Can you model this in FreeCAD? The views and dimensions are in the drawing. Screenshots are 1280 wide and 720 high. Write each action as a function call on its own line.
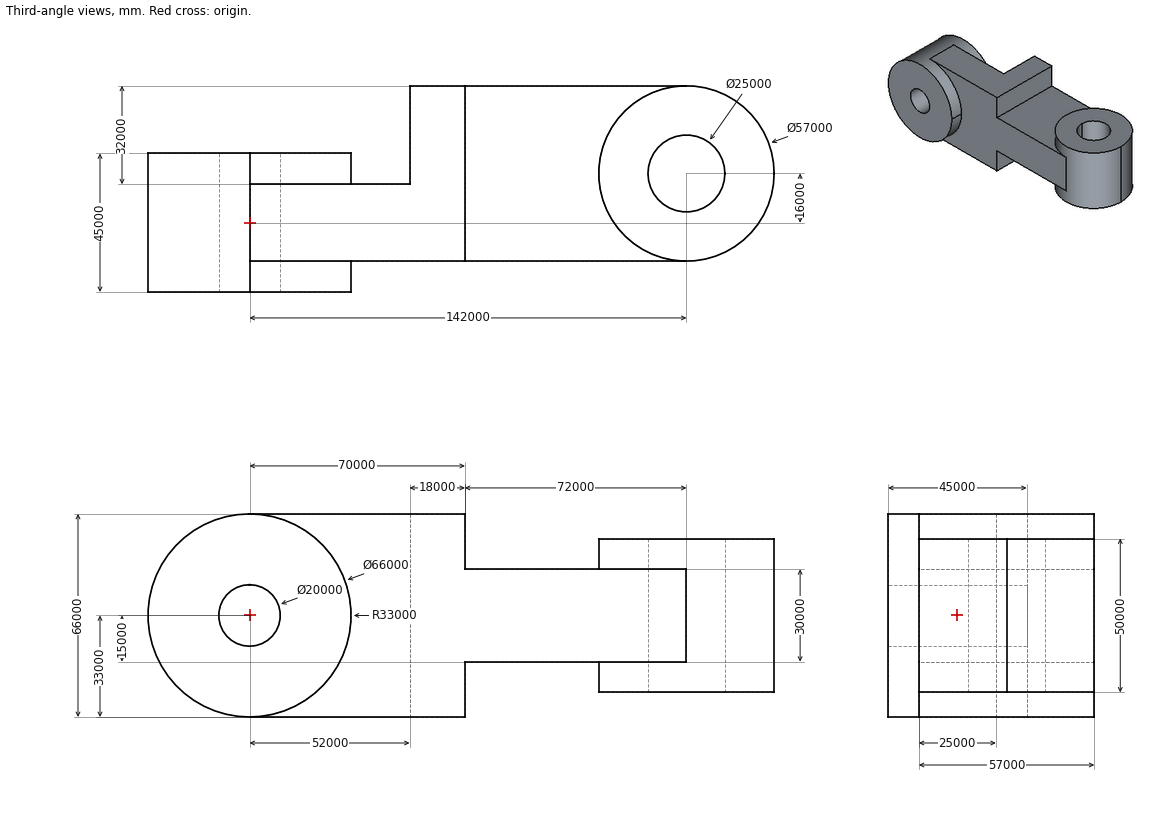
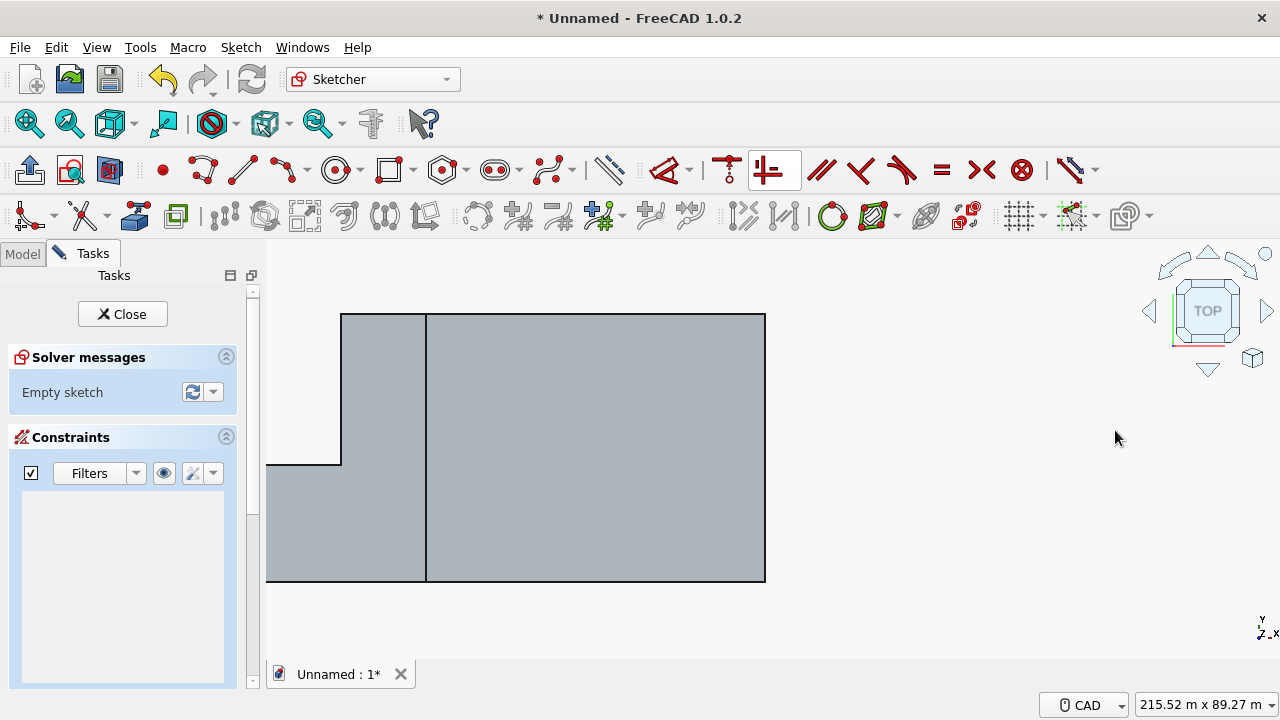
click(336, 170)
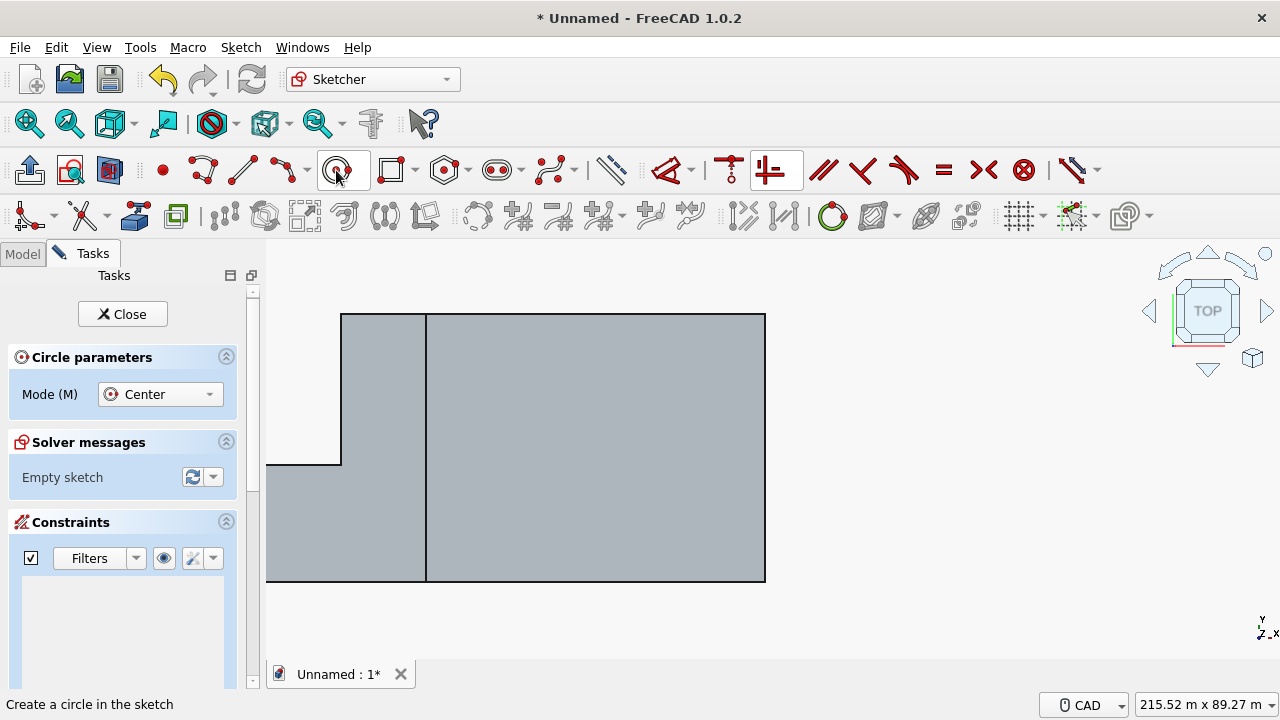
click(765, 448)
click(859, 353)
key(Escape)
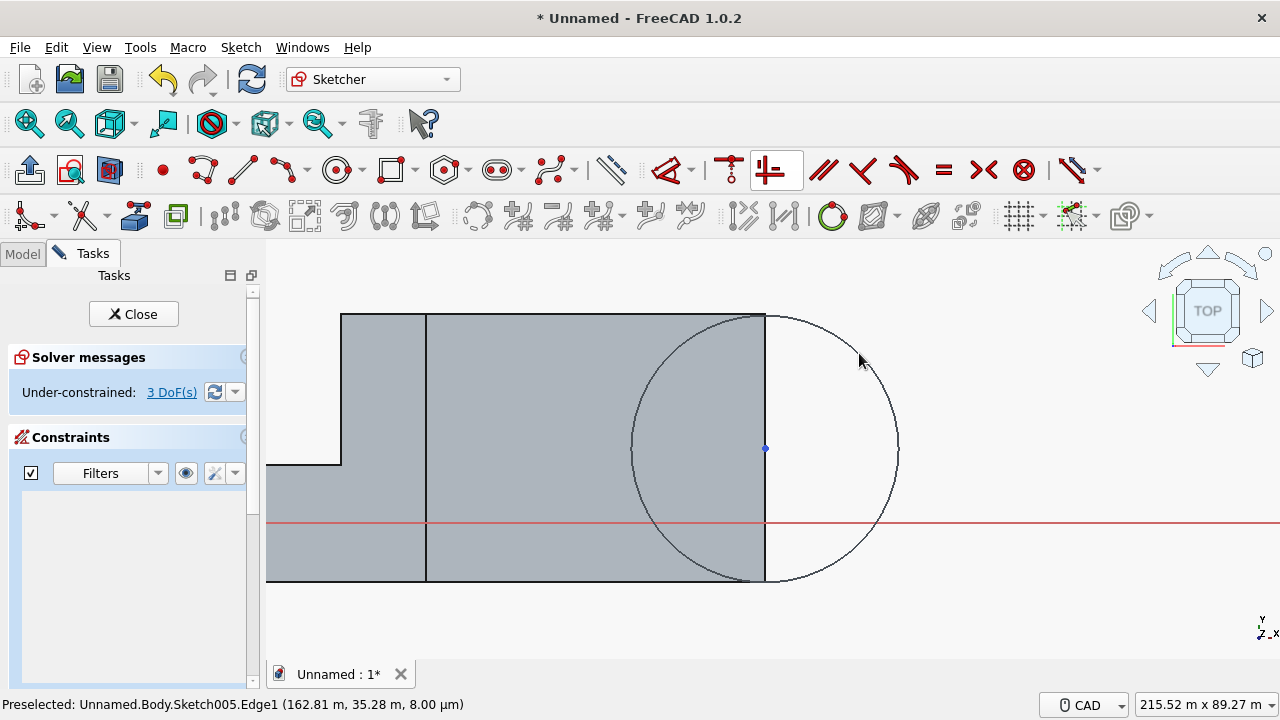
key(d)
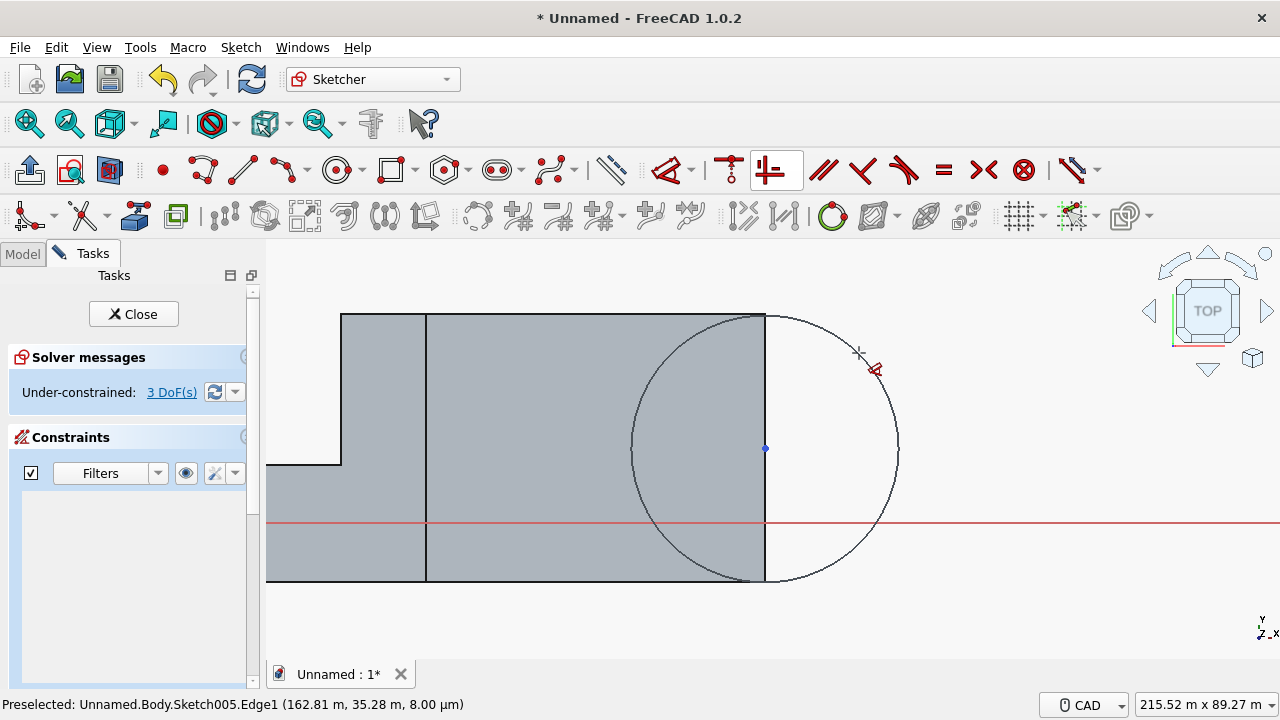
click(859, 354)
click(882, 331)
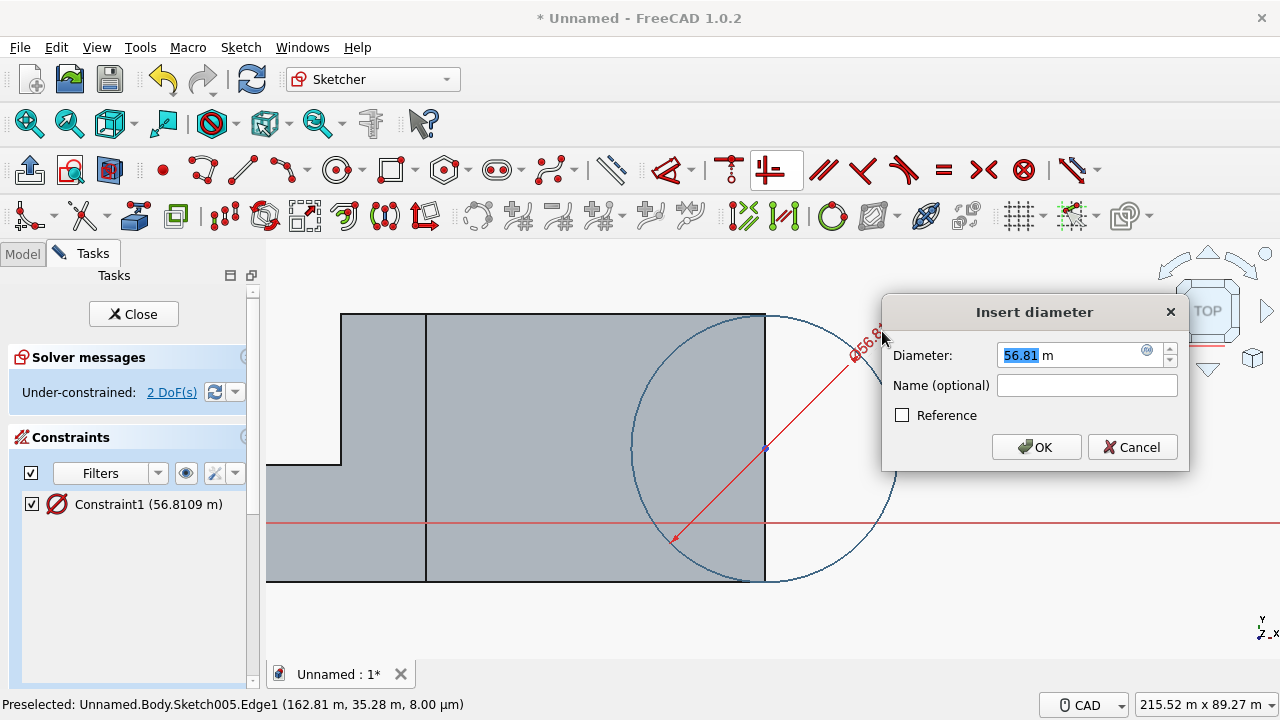
key(ctrl+a)
text(57000 mm)
key(Return)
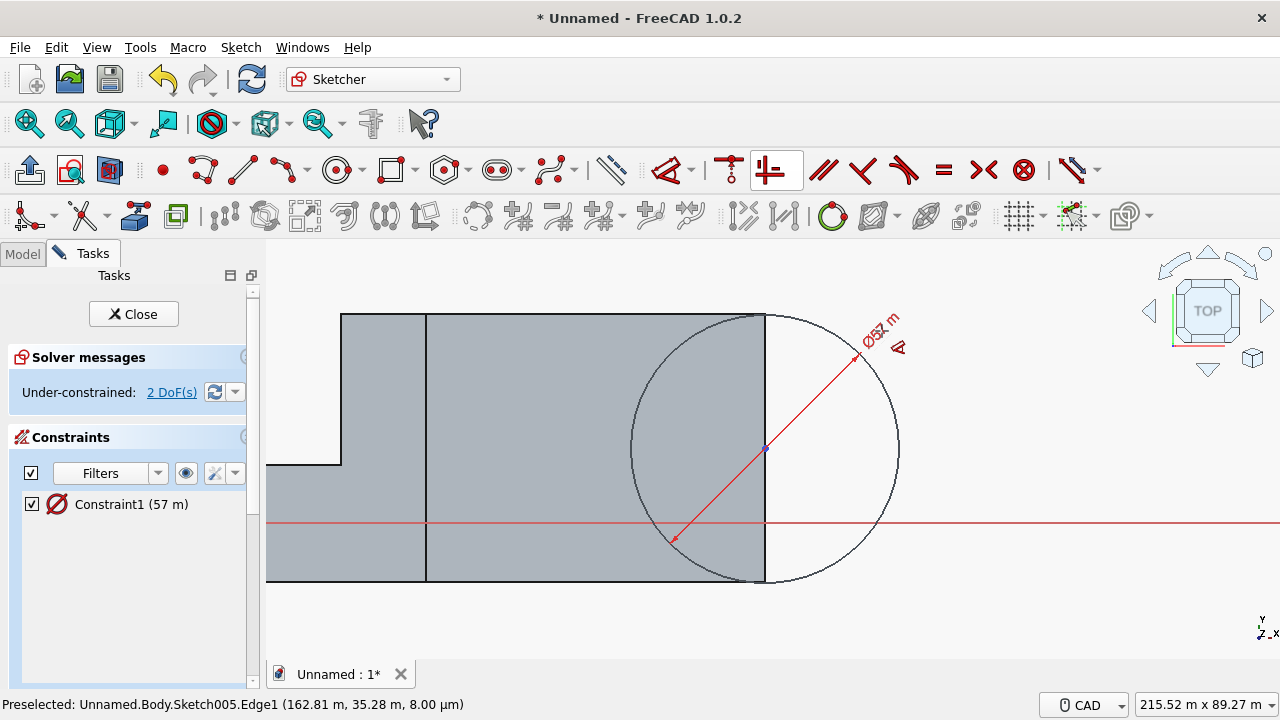
click(765, 449)
click(799, 486)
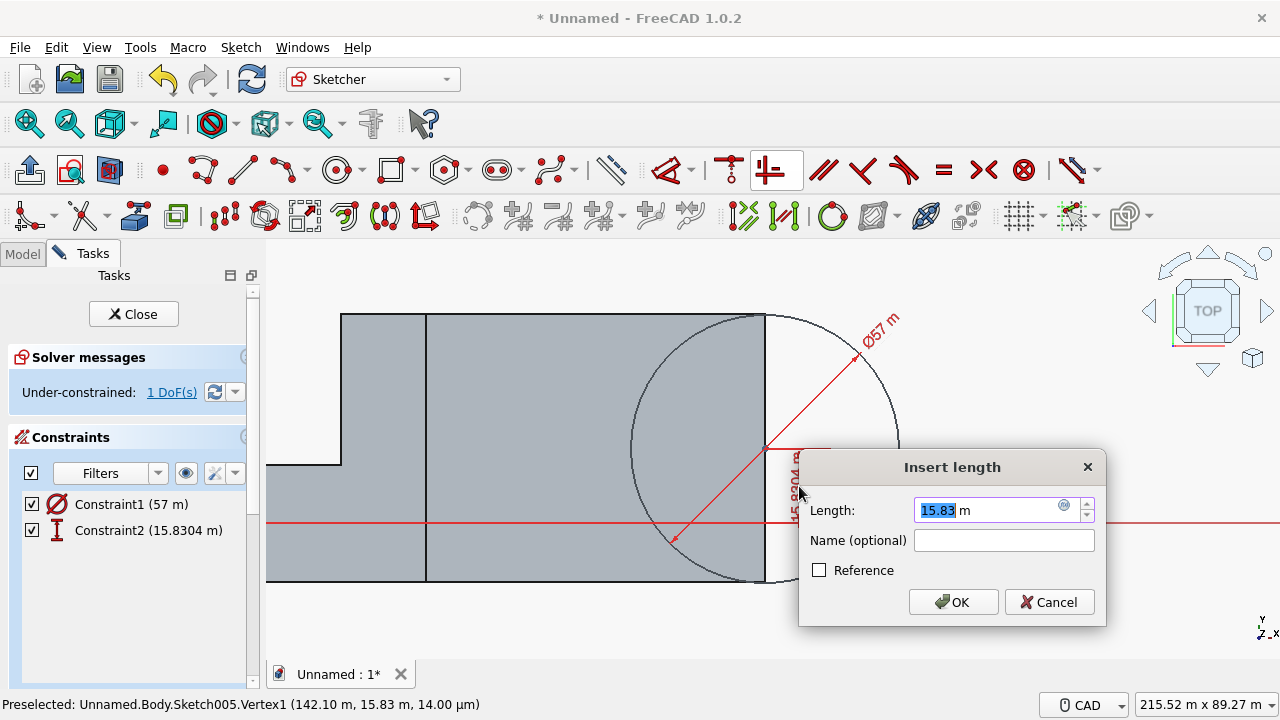
key(ctrl+a)
text(16000 mm)
key(Return)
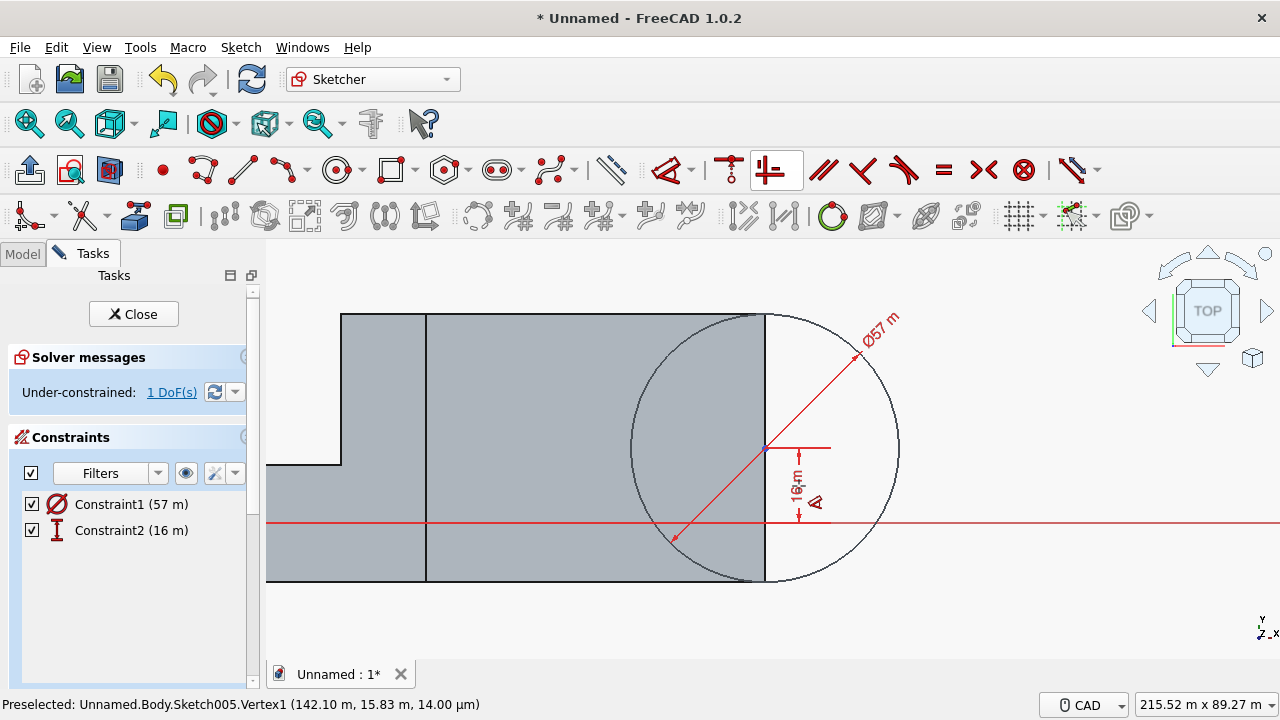
click(765, 448)
click(530, 557)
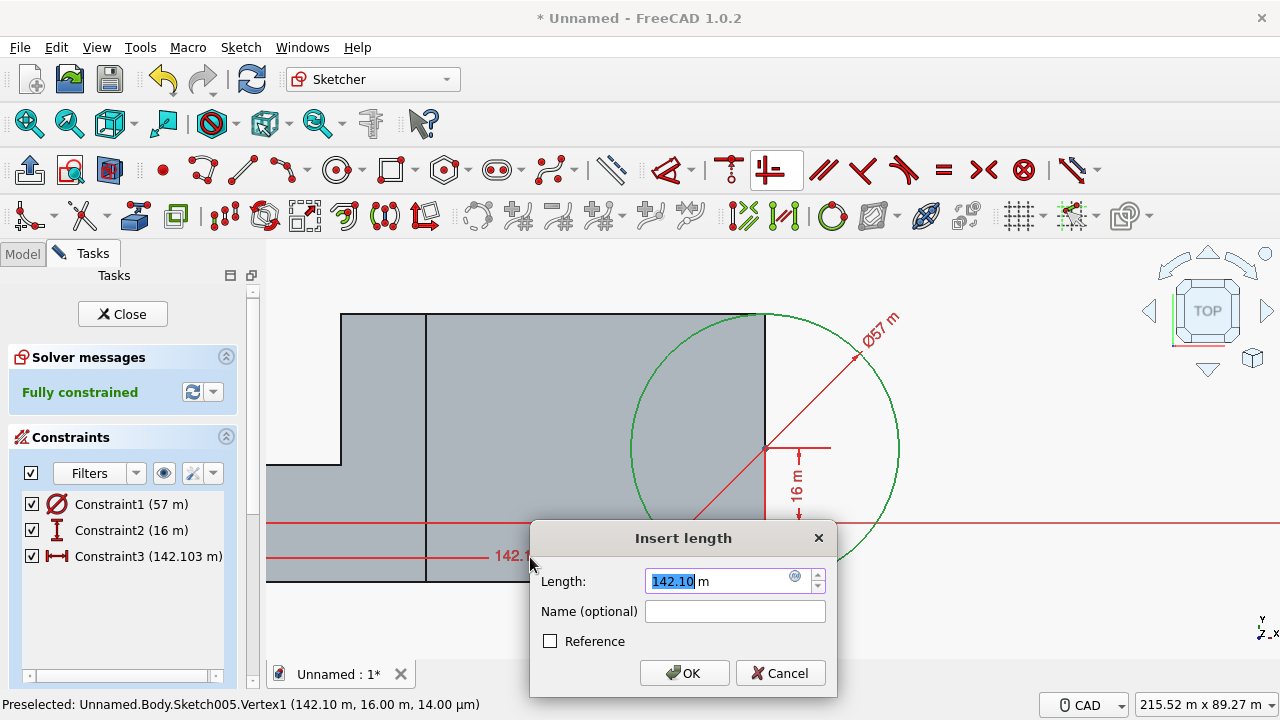
key(ctrl+a)
text(142000 mm)
key(Return)
key(Escape)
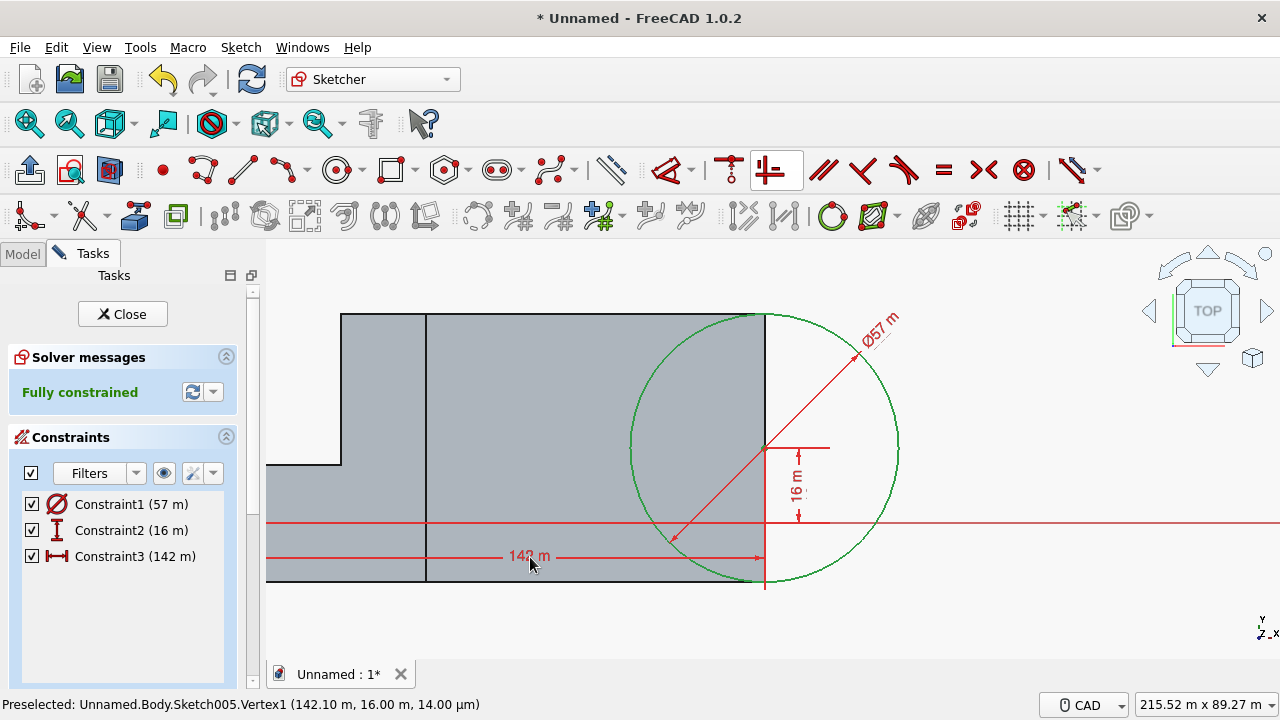
click(123, 314)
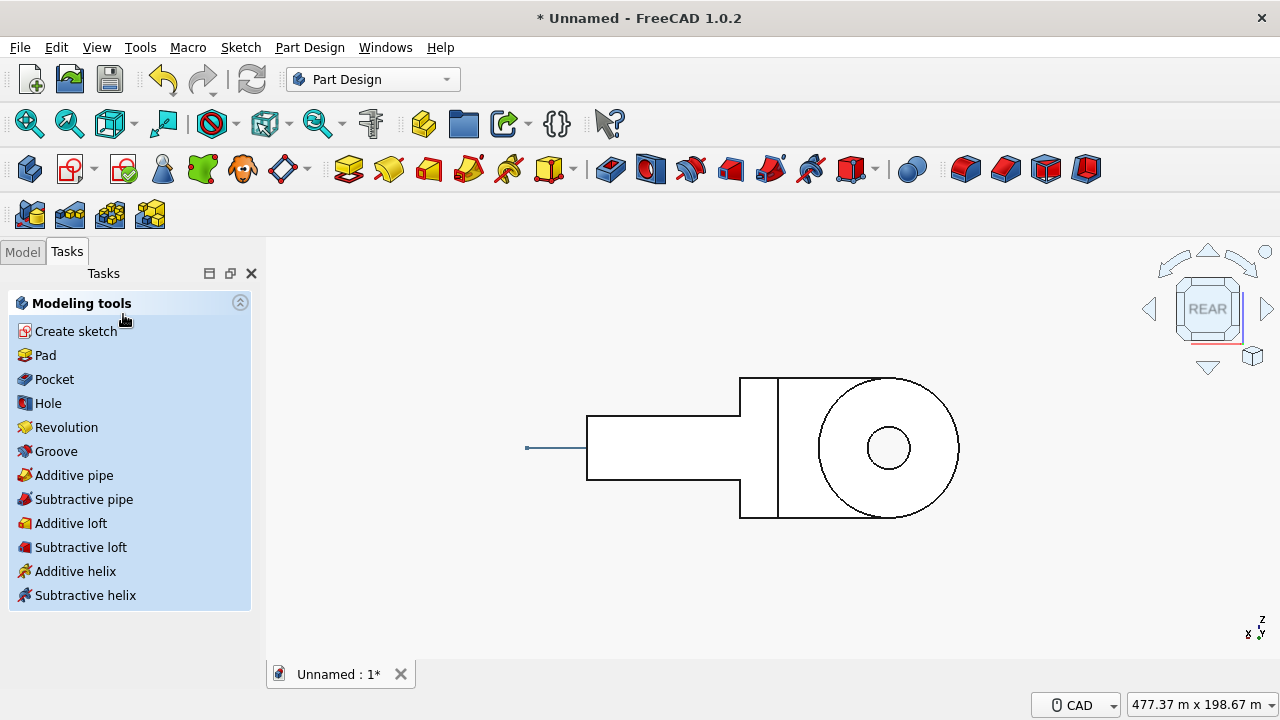
click(350, 170)